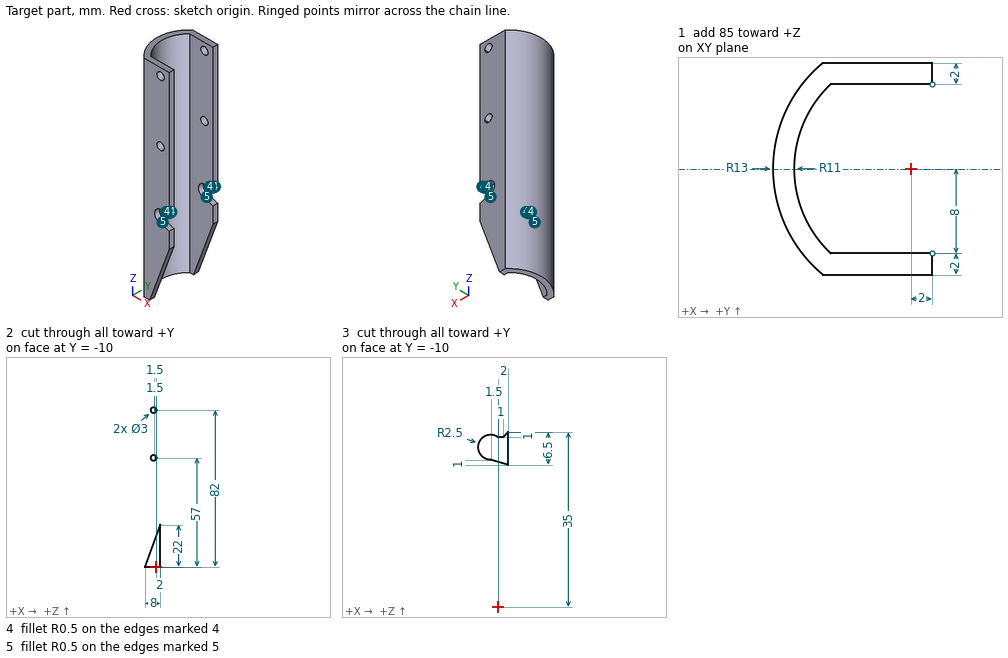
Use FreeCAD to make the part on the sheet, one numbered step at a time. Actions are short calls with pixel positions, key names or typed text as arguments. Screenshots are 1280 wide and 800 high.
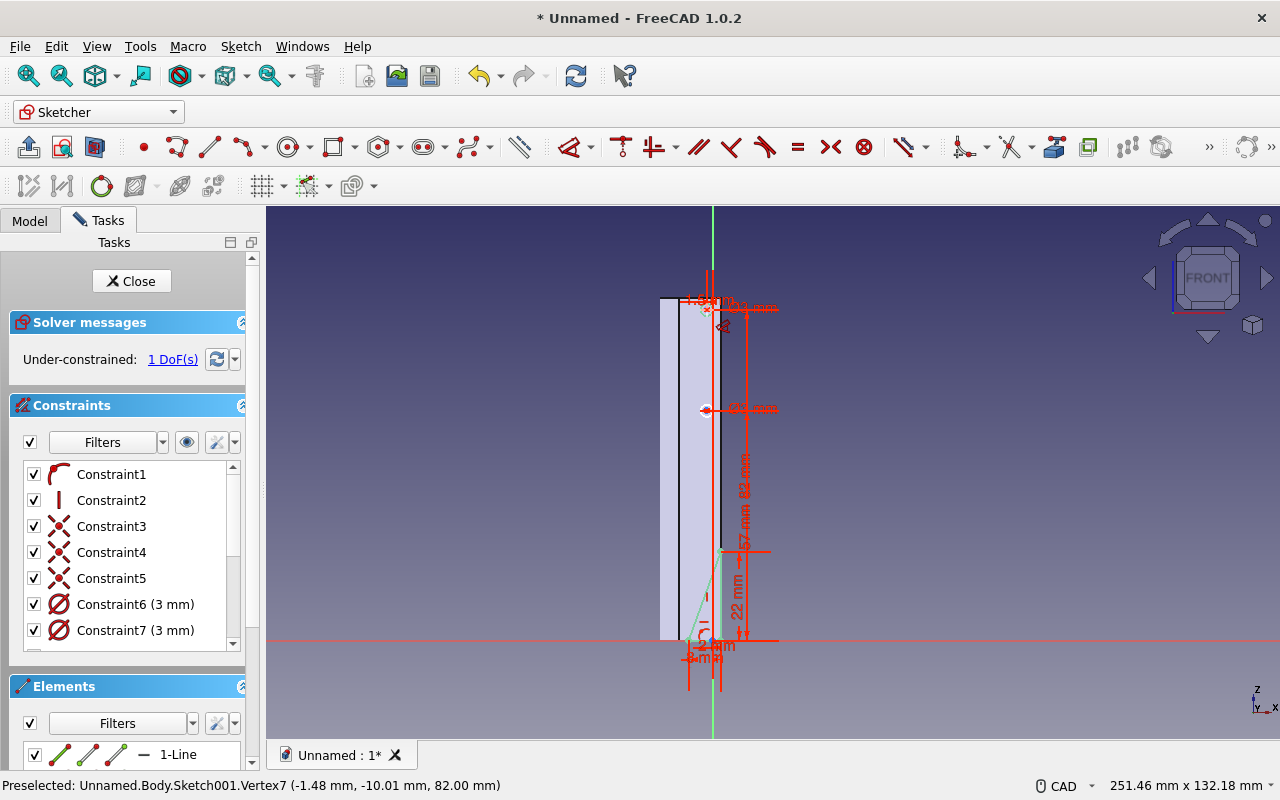
scroll(707, 411, up, 10)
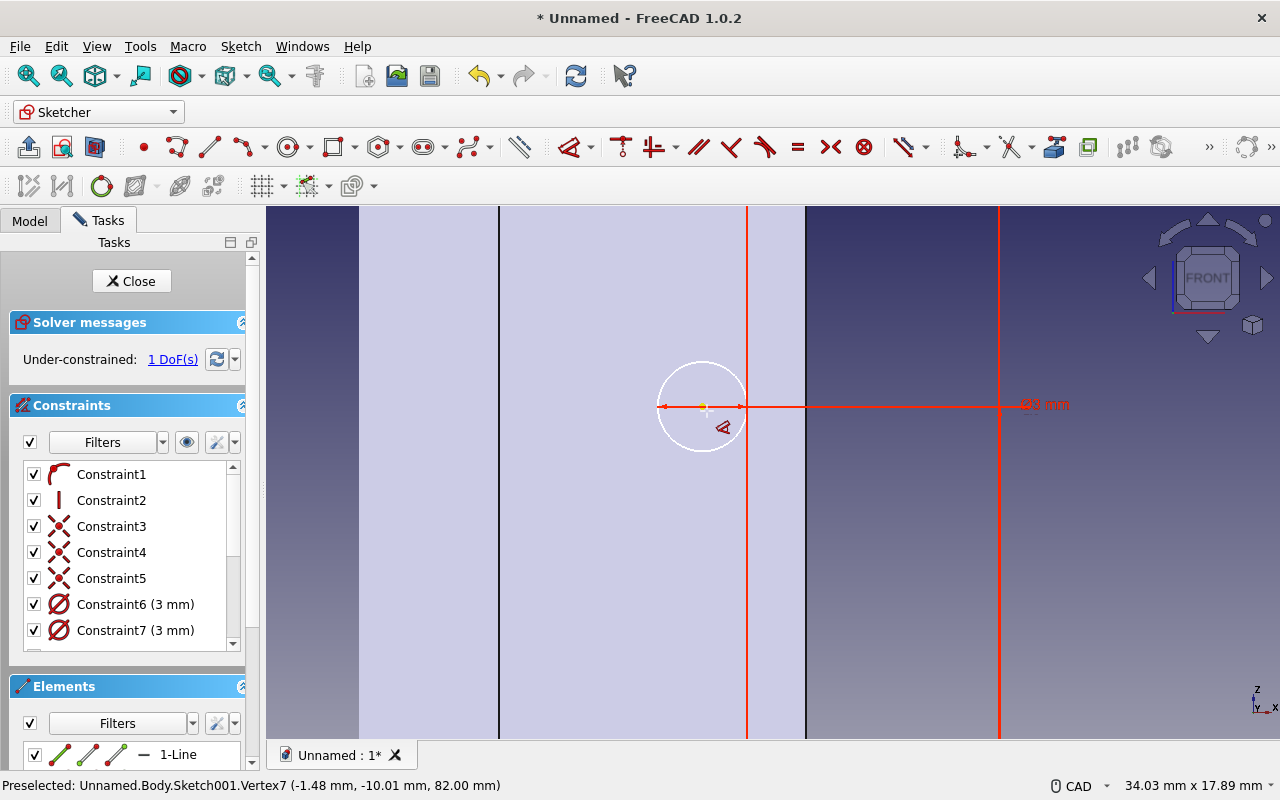
click(703, 407)
click(725, 349)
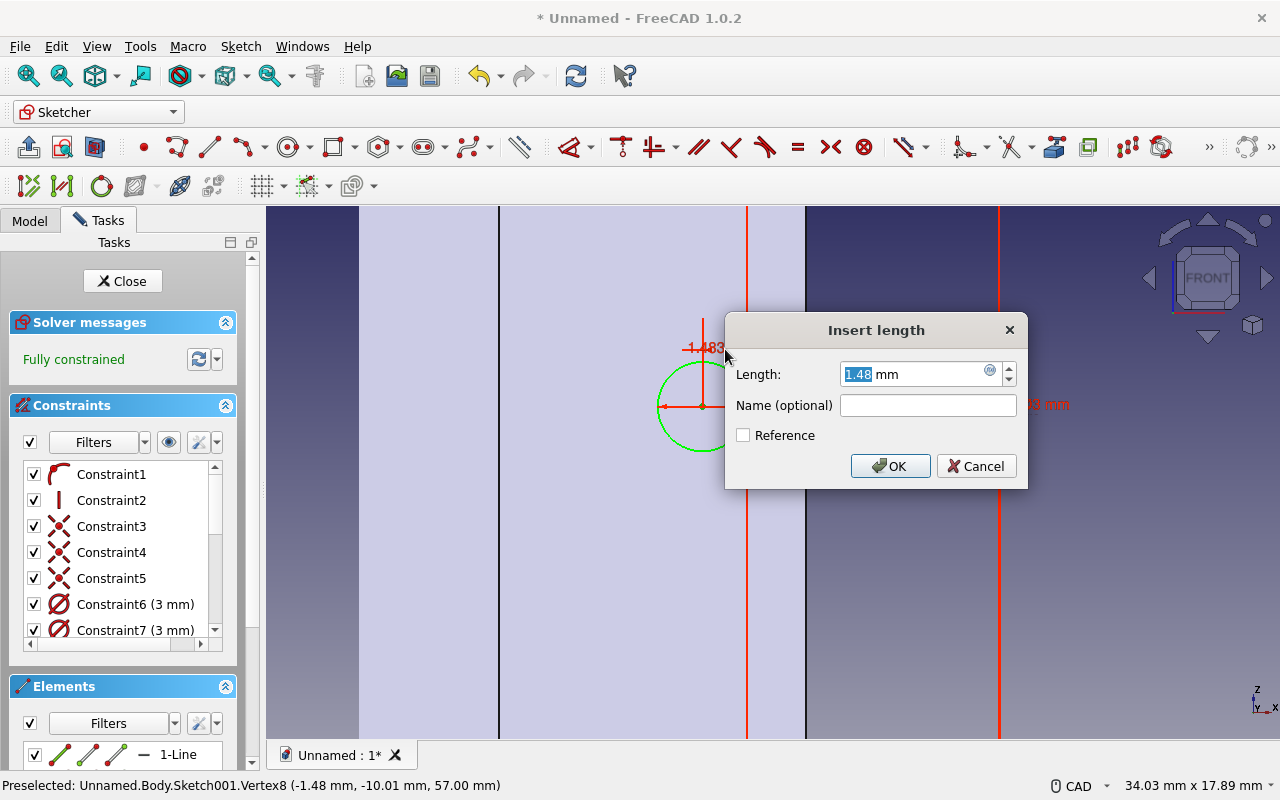
text(1.5)
key(Return)
key(Escape)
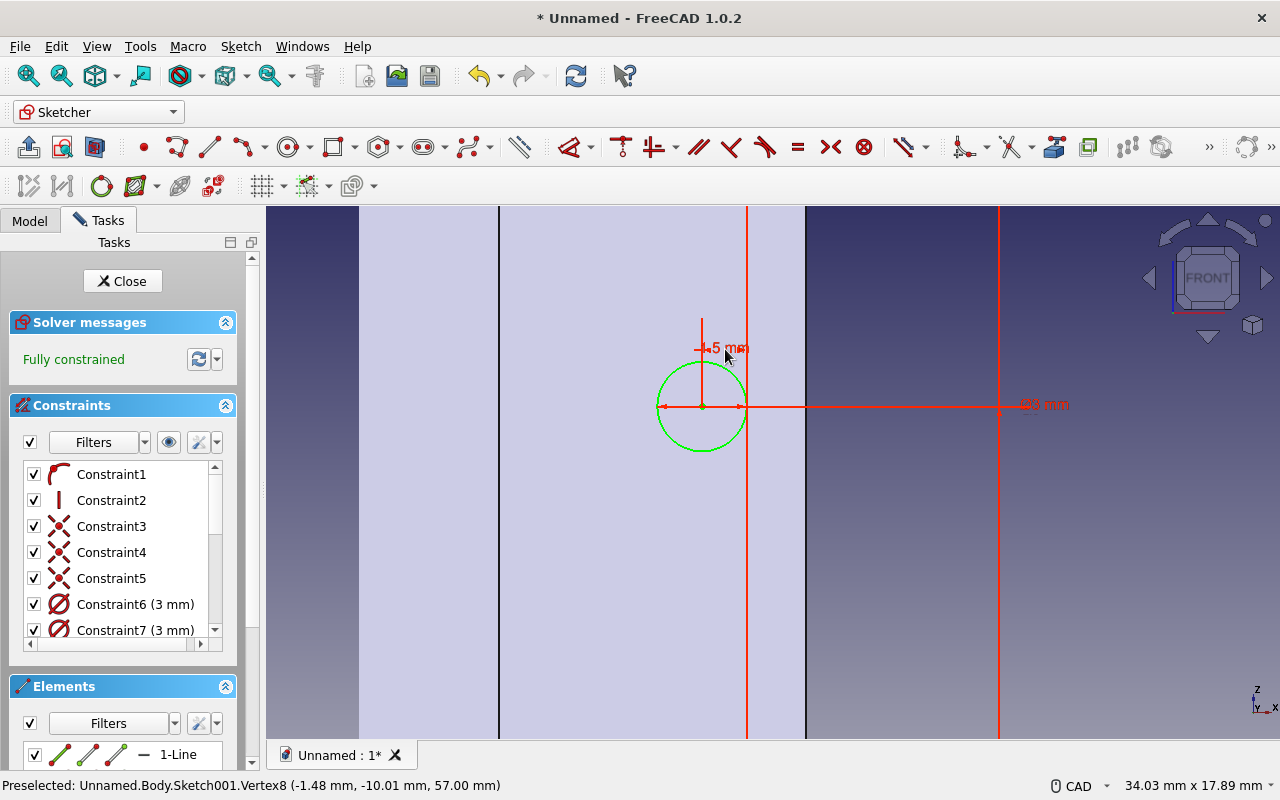
click(123, 281)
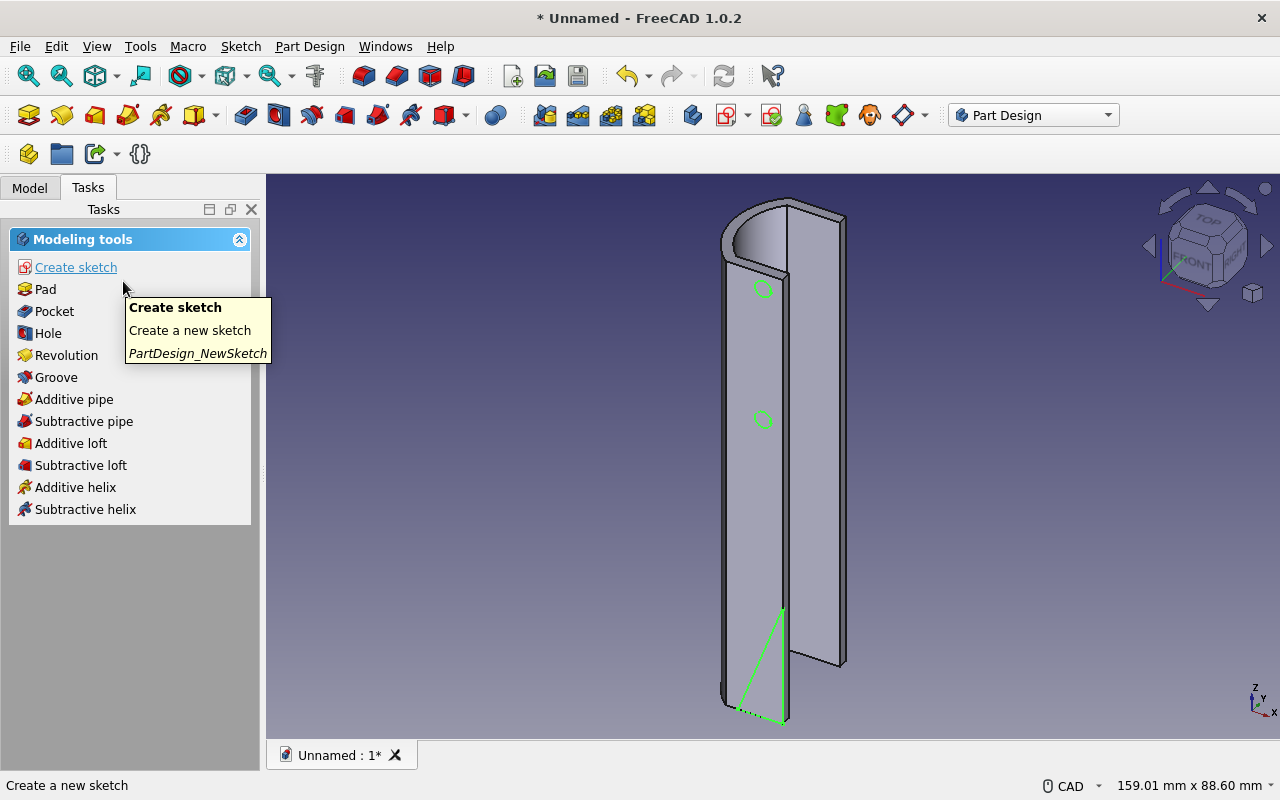
click(246, 116)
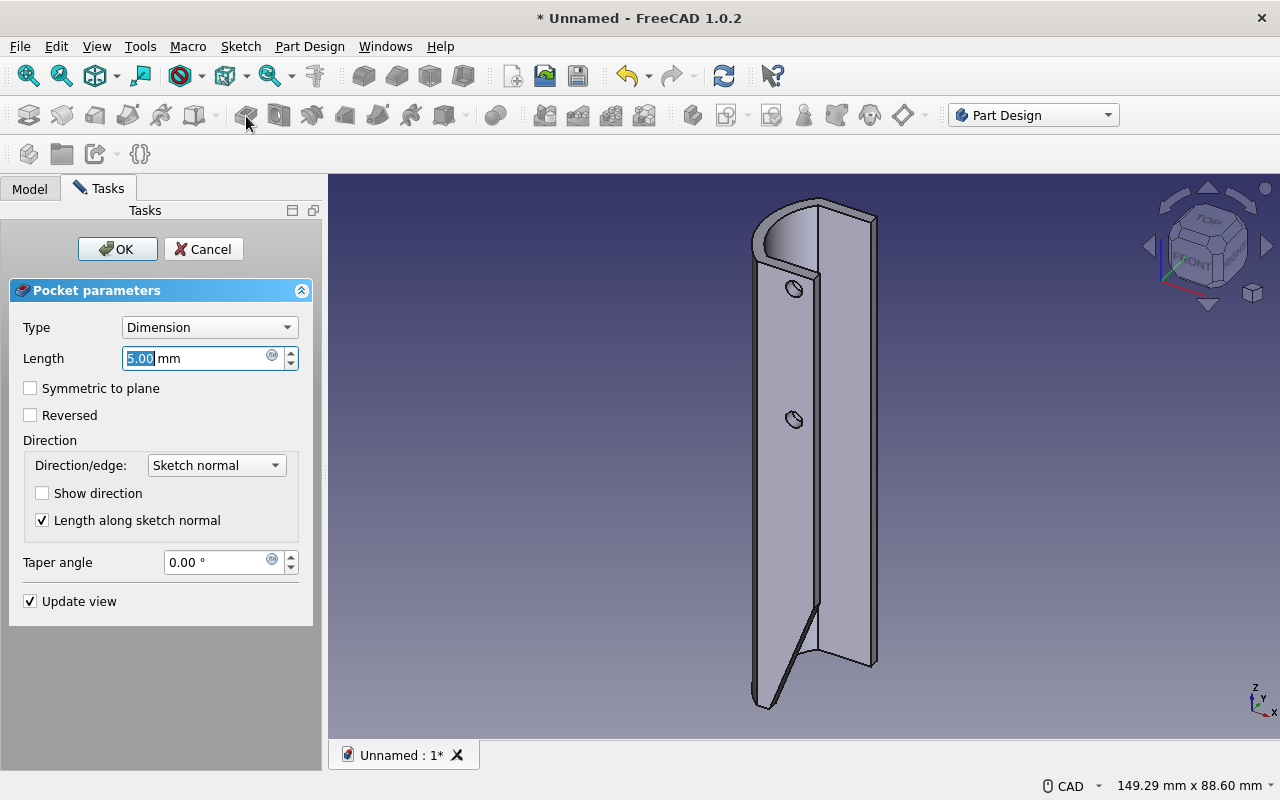
click(210, 328)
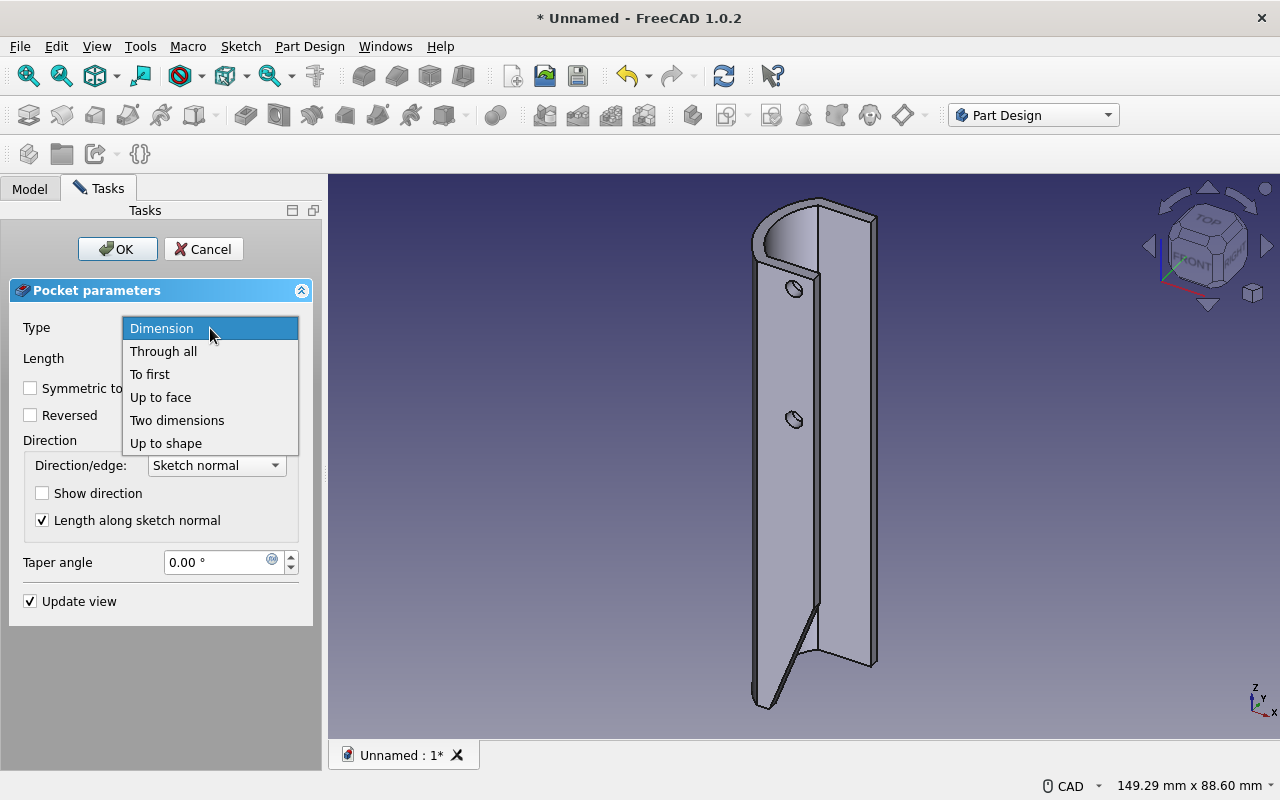
click(208, 352)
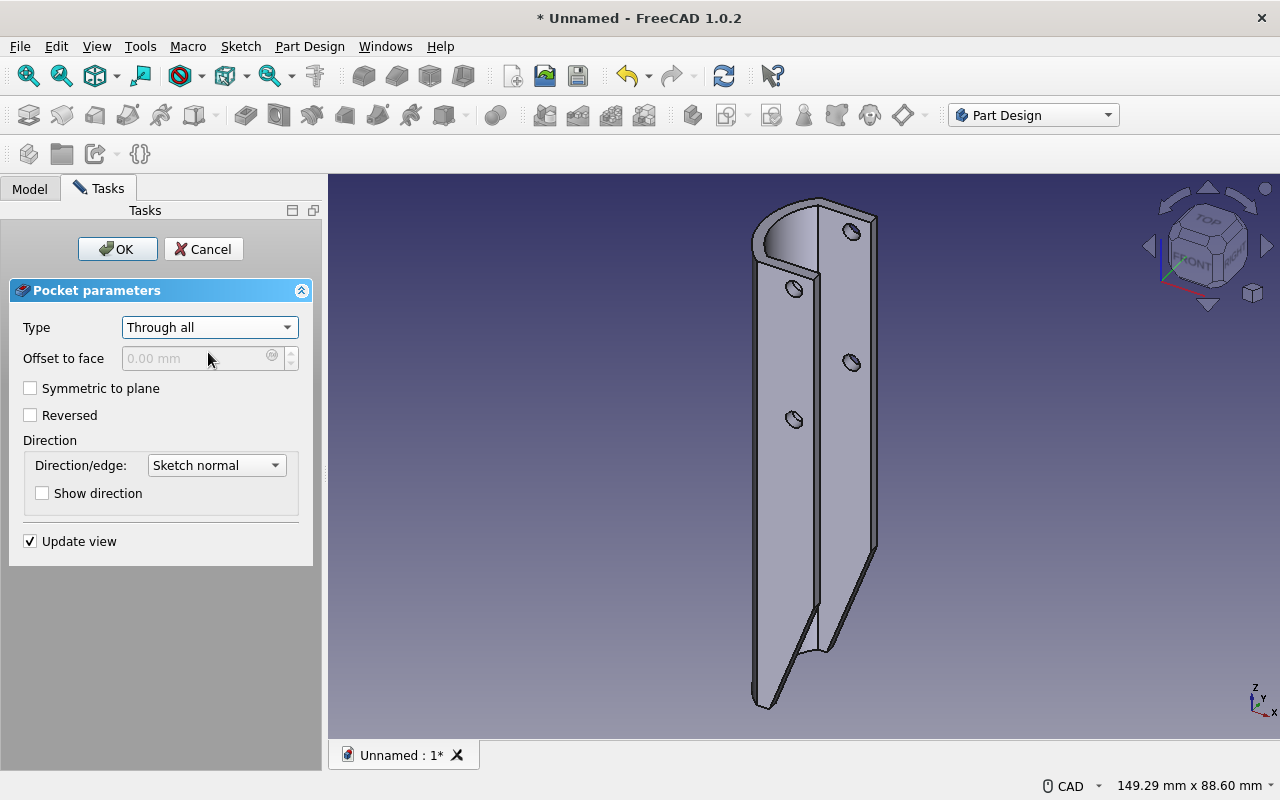
click(118, 249)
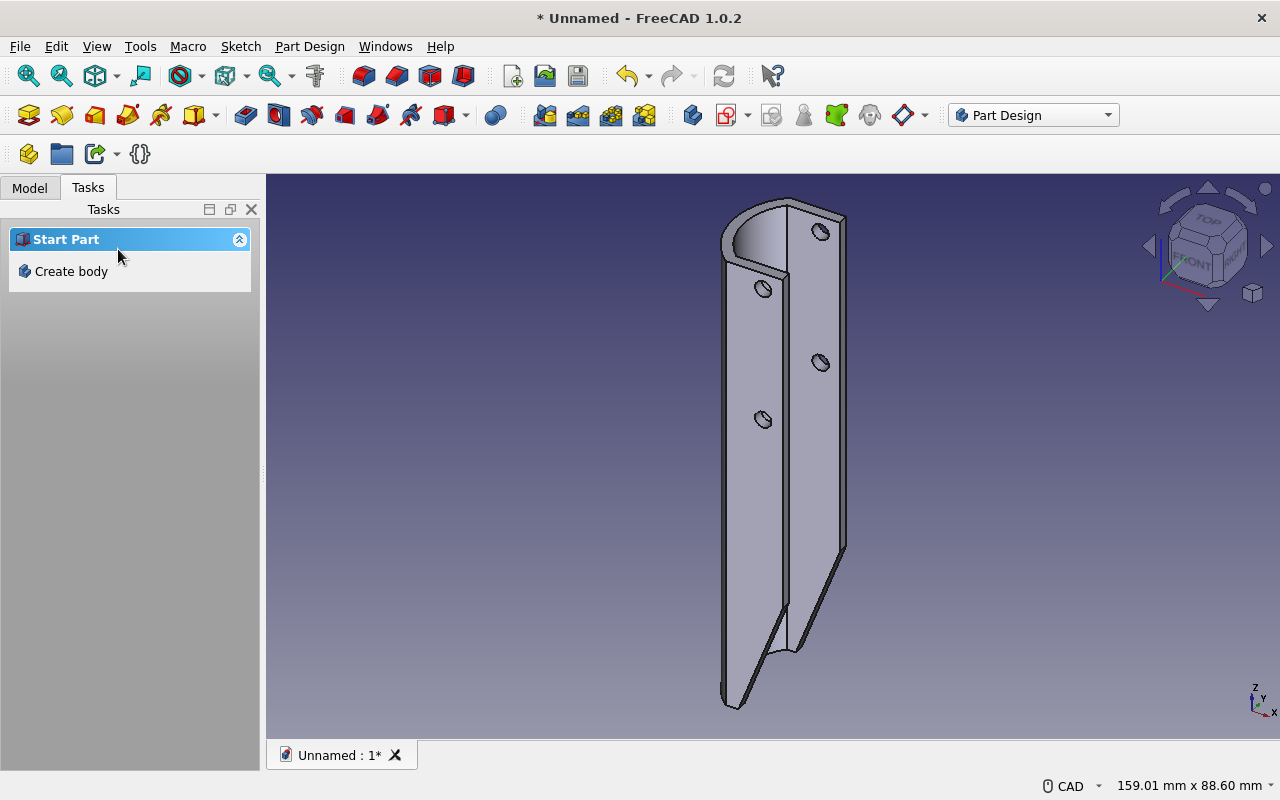
click(754, 365)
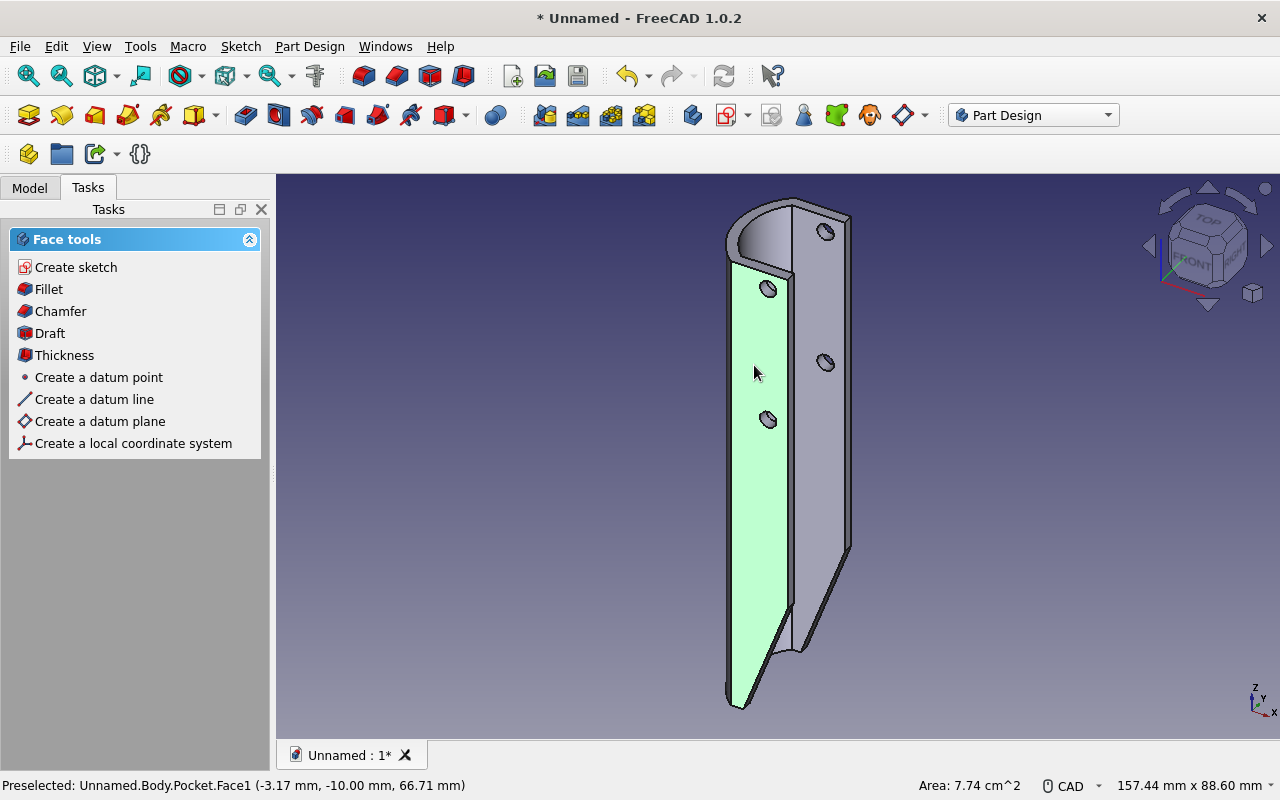
click(726, 116)